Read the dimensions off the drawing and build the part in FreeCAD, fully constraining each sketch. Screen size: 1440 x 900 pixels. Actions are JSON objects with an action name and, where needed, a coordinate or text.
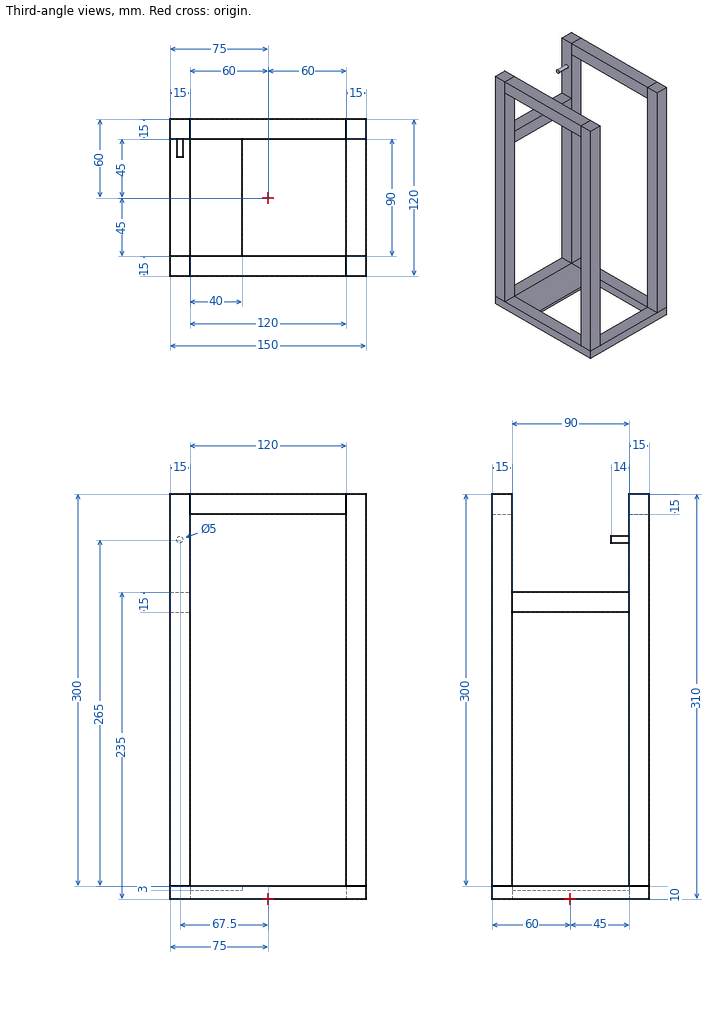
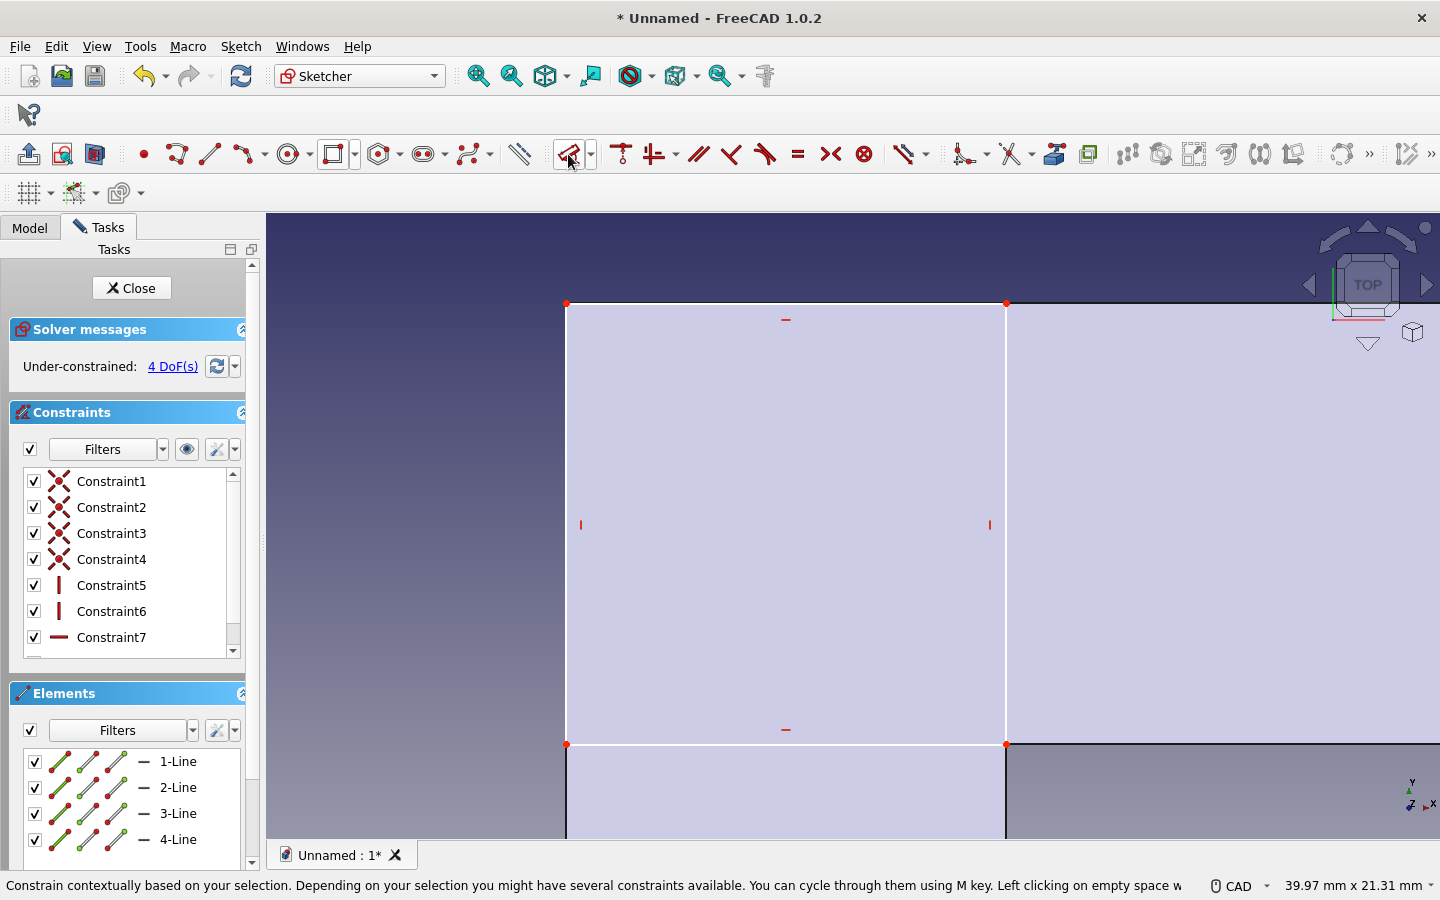
{"action": "left_click", "coordinate": [566, 436]}
{"action": "left_click", "coordinate": [532, 524]}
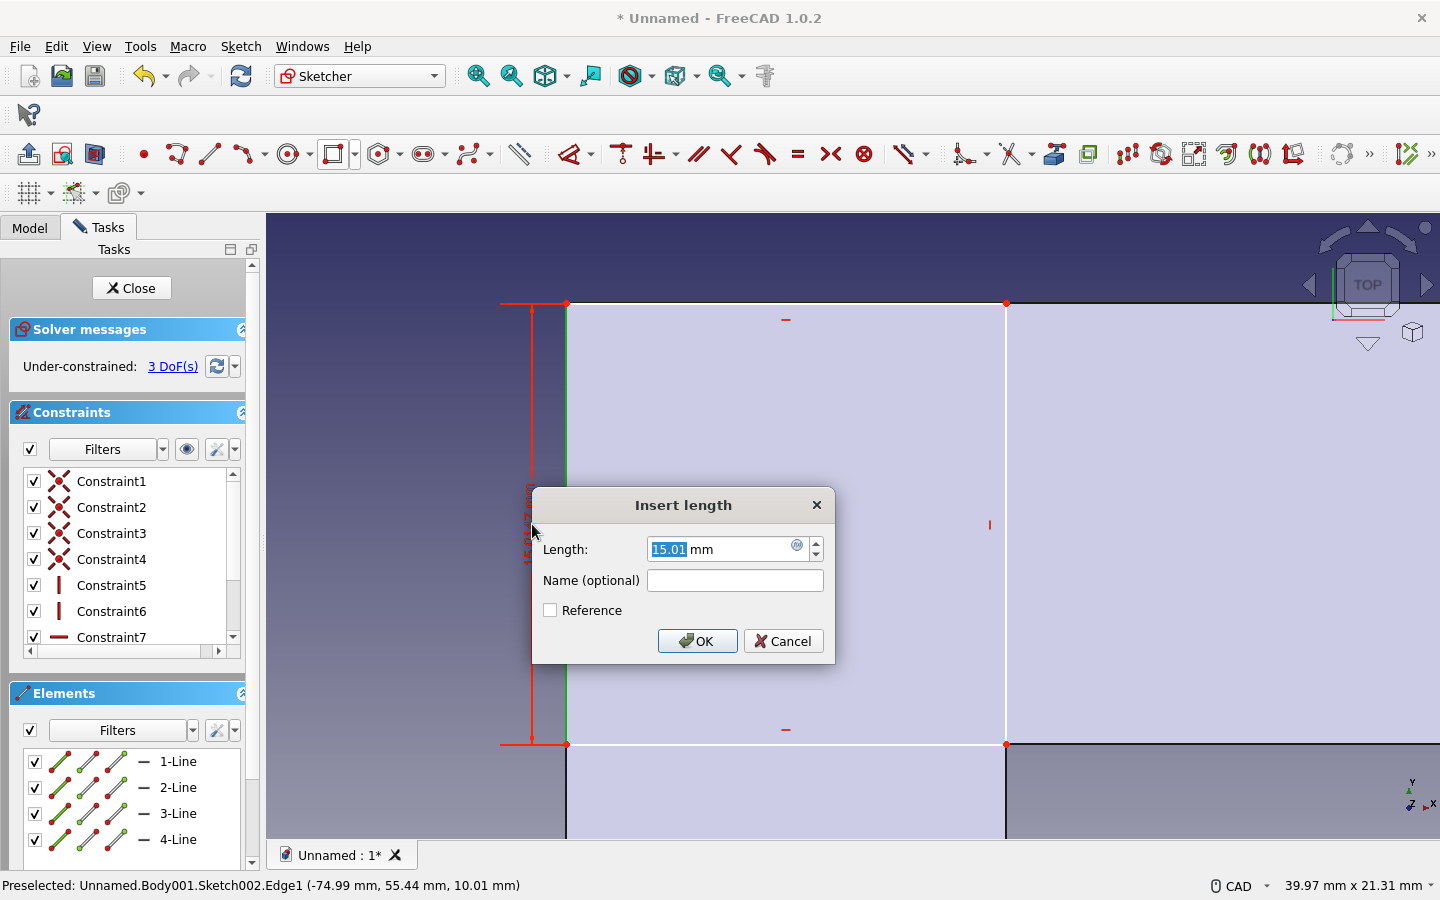
{"action": "type", "text": "15"}
{"action": "key", "text": "Return"}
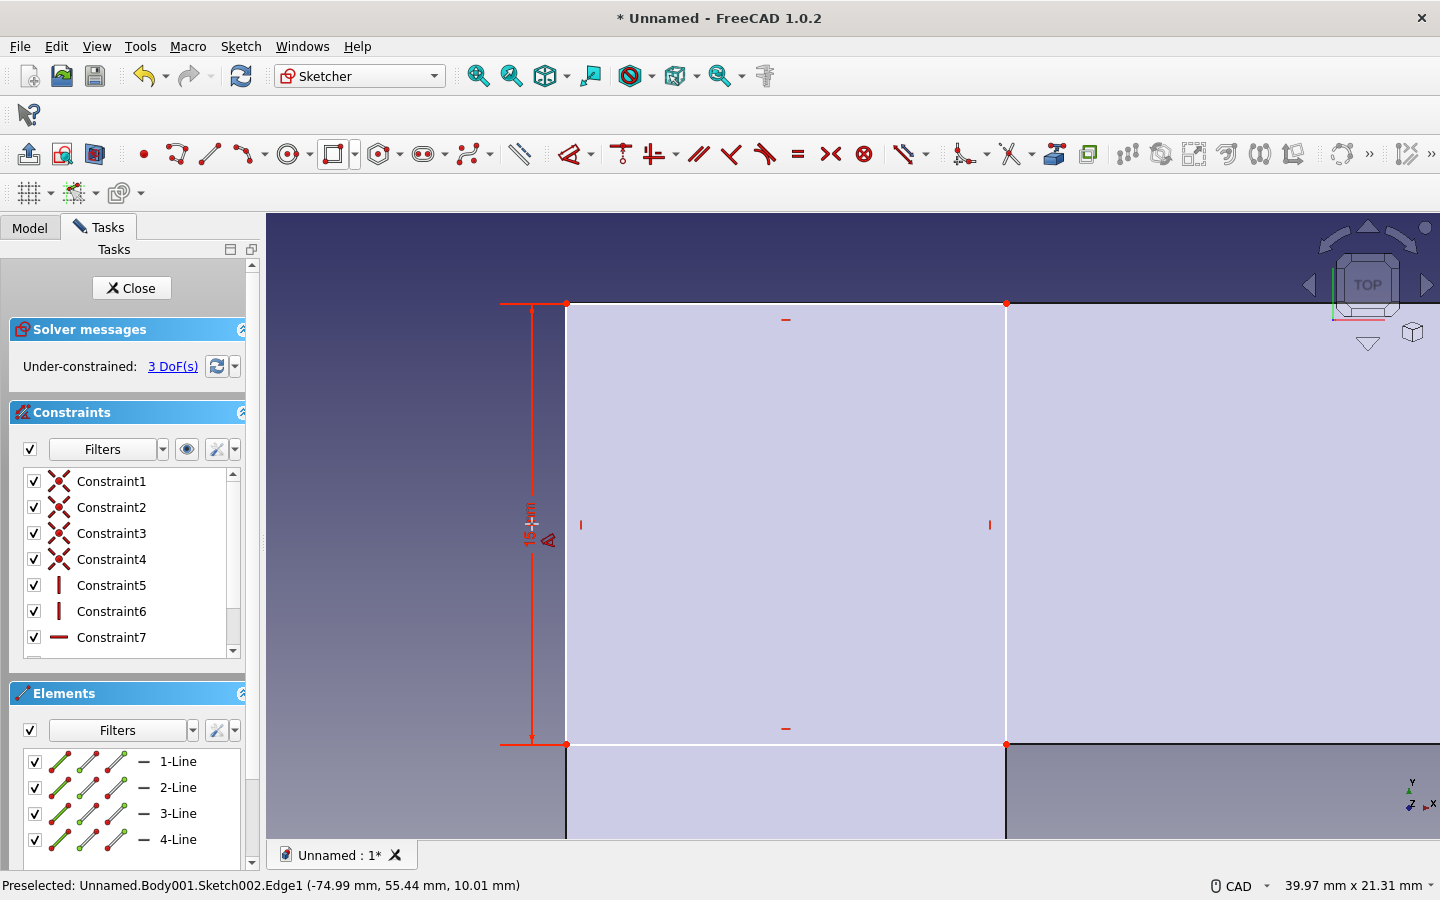
{"action": "left_click", "coordinate": [698, 745]}
{"action": "left_click", "coordinate": [786, 779]}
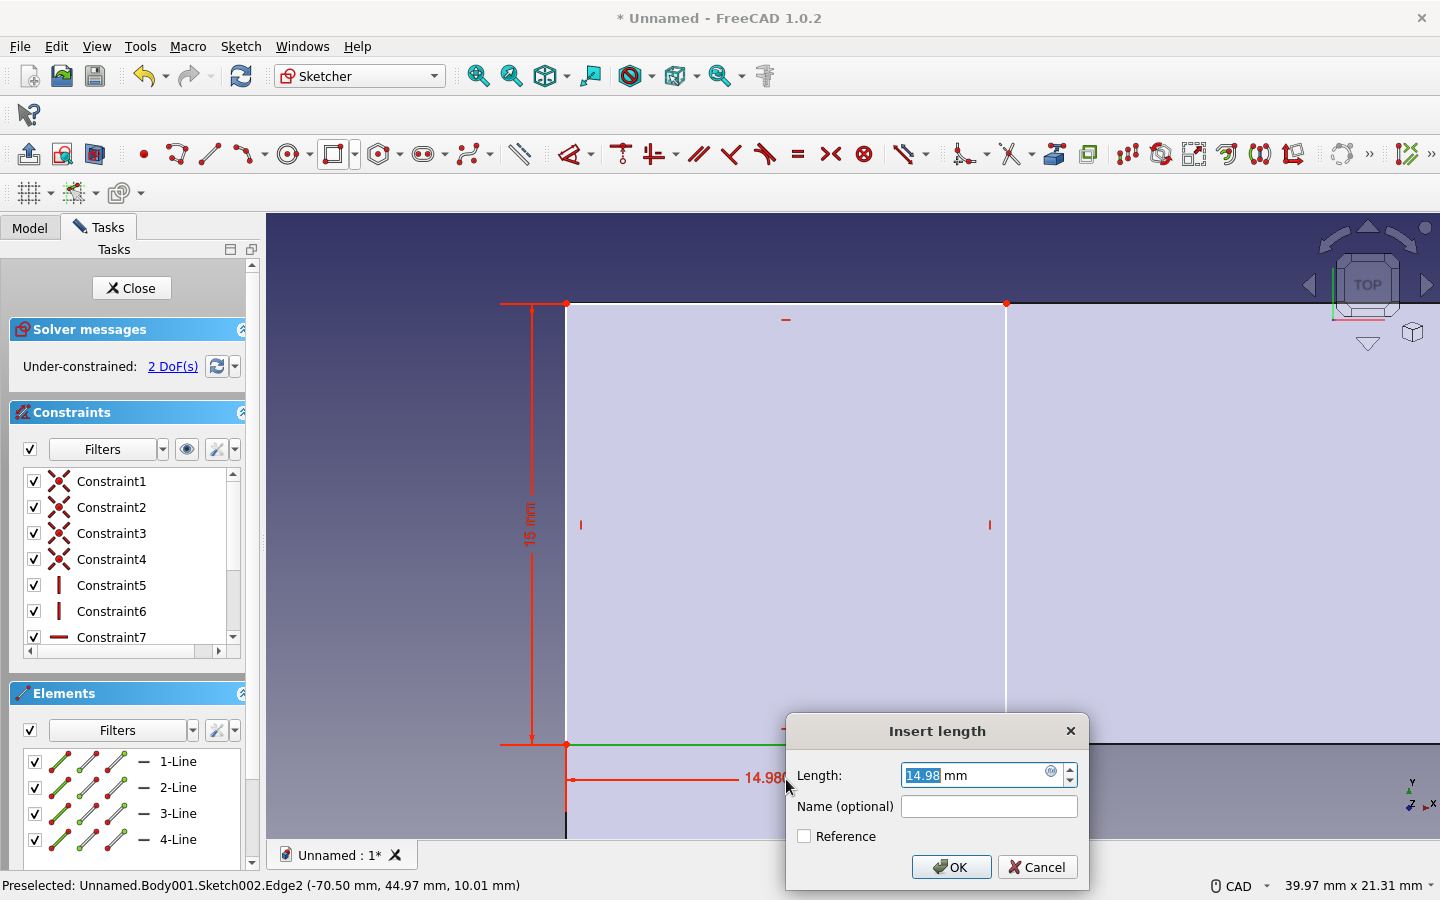
{"action": "type", "text": "15"}
{"action": "key", "text": "Return"}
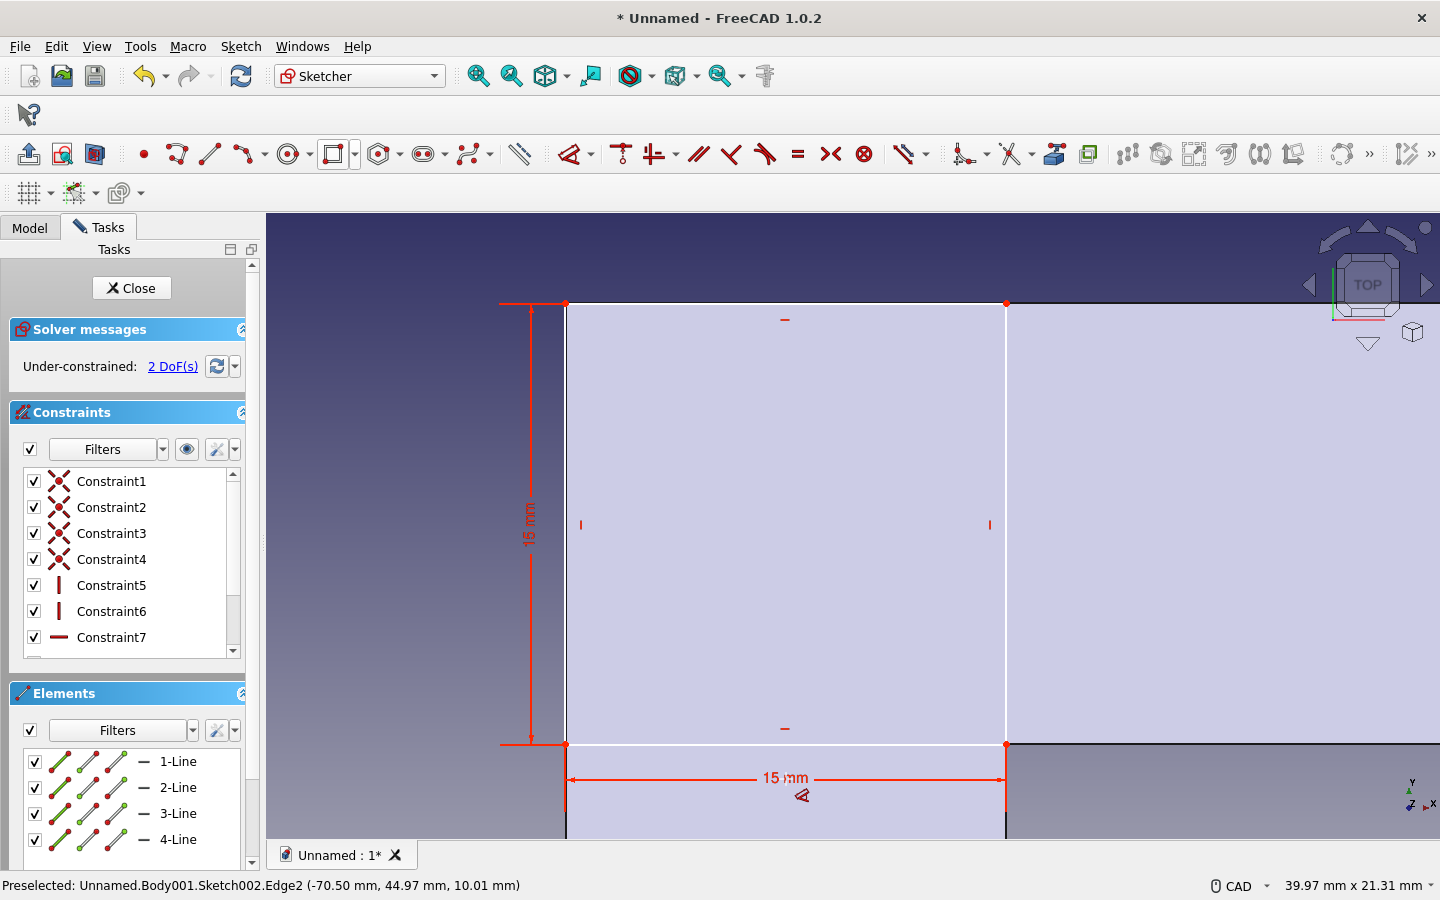
{"action": "left_click", "coordinate": [565, 304]}
{"action": "left_click", "coordinate": [920, 270]}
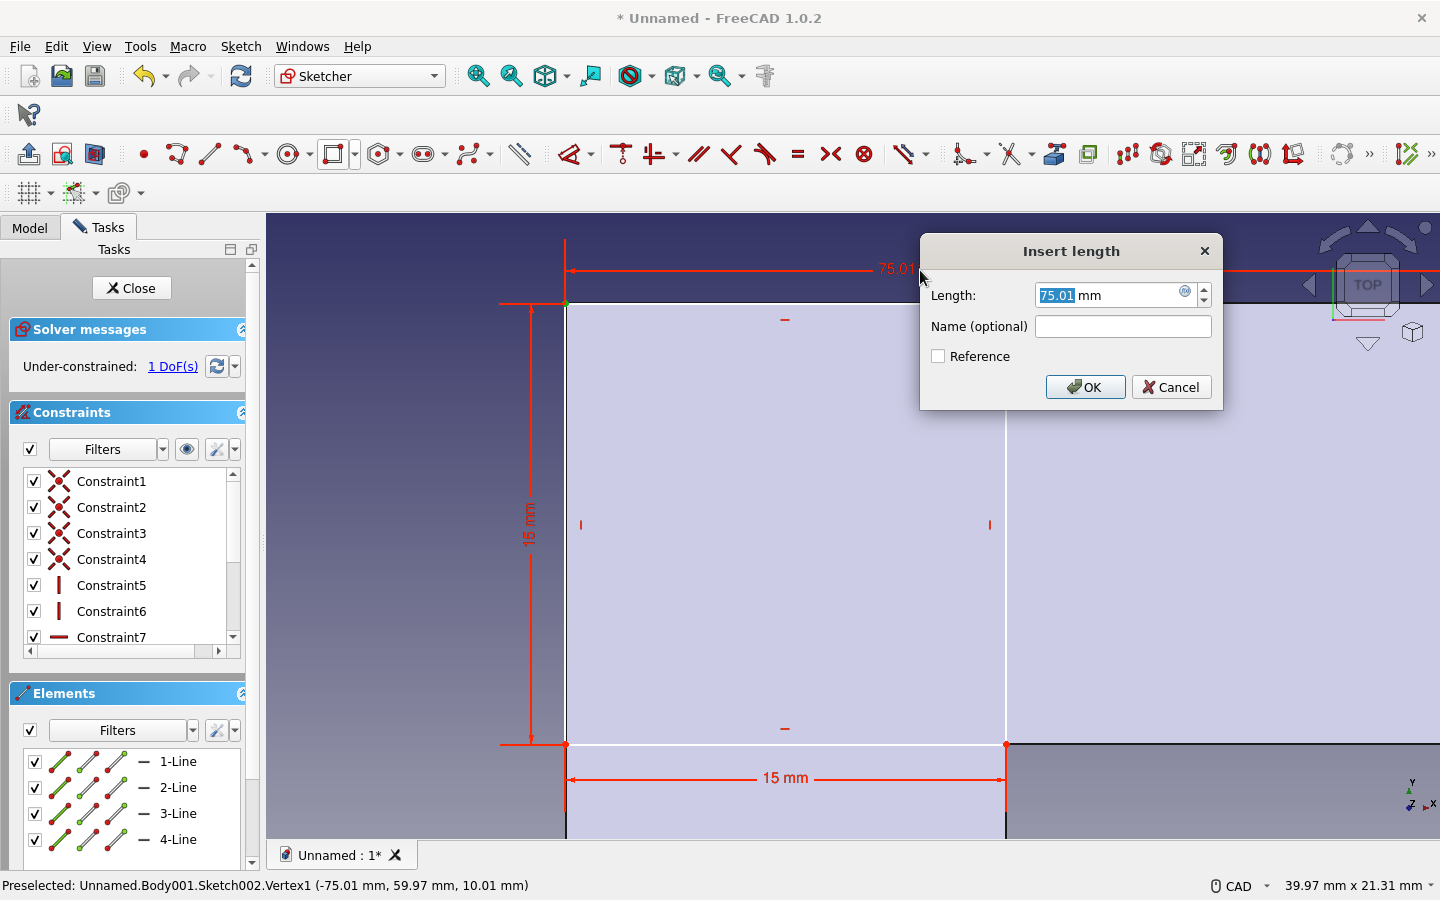
{"action": "type", "text": "75"}
{"action": "key", "text": "Return"}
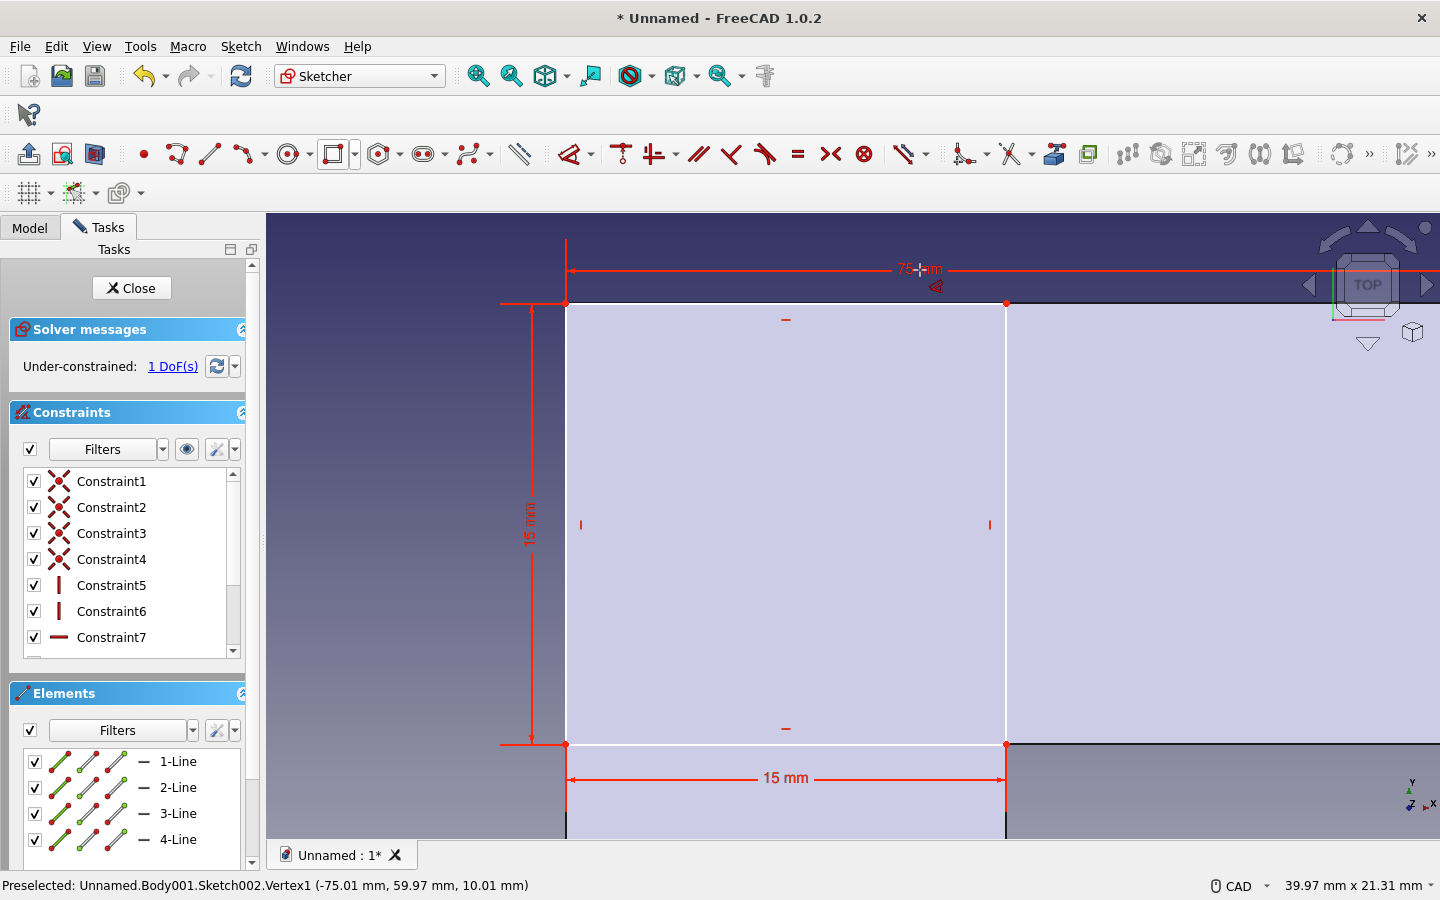
{"action": "left_click", "coordinate": [566, 304]}
{"action": "left_click", "coordinate": [532, 557]}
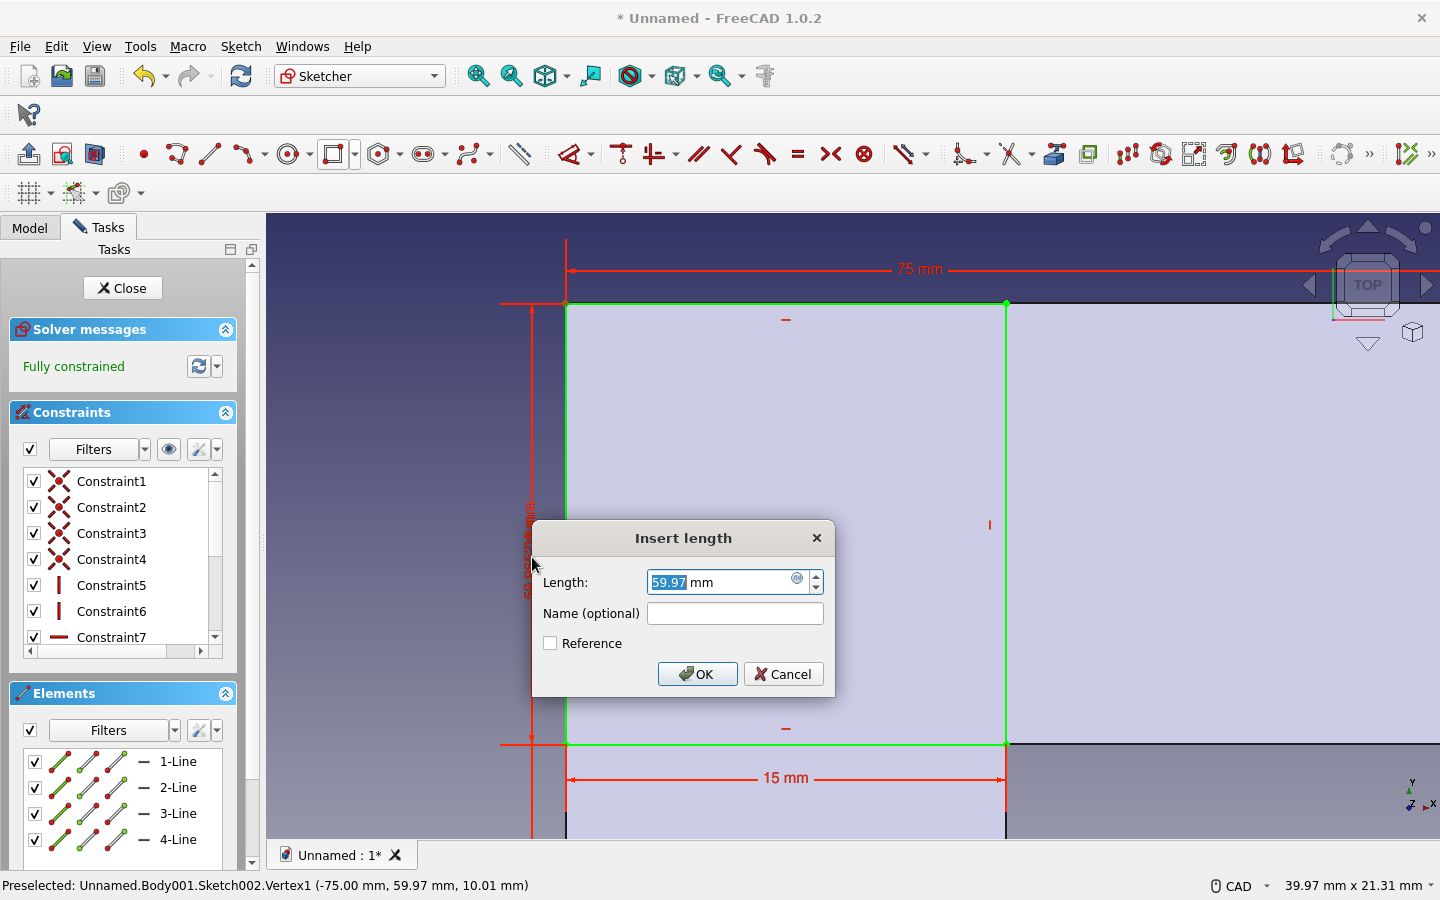
{"action": "type", "text": "60"}
{"action": "key", "text": "Return"}
{"action": "key", "text": "Escape"}